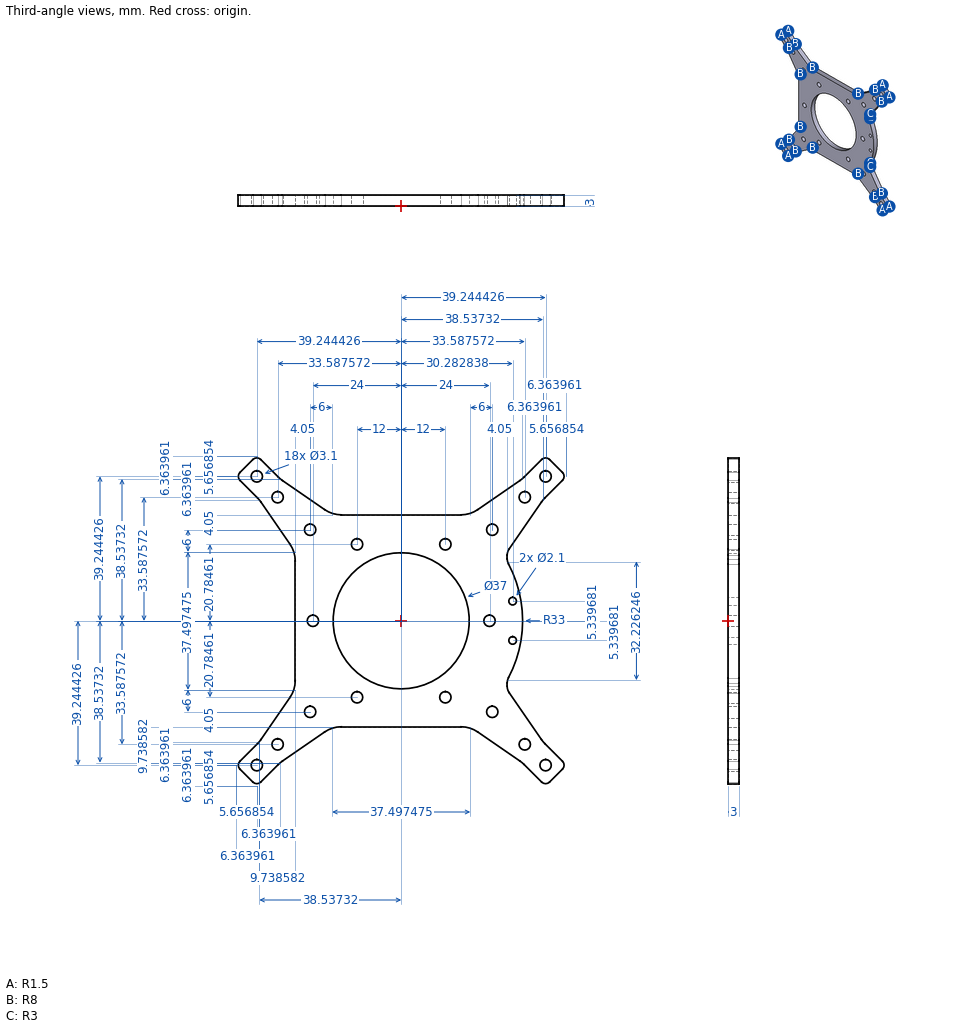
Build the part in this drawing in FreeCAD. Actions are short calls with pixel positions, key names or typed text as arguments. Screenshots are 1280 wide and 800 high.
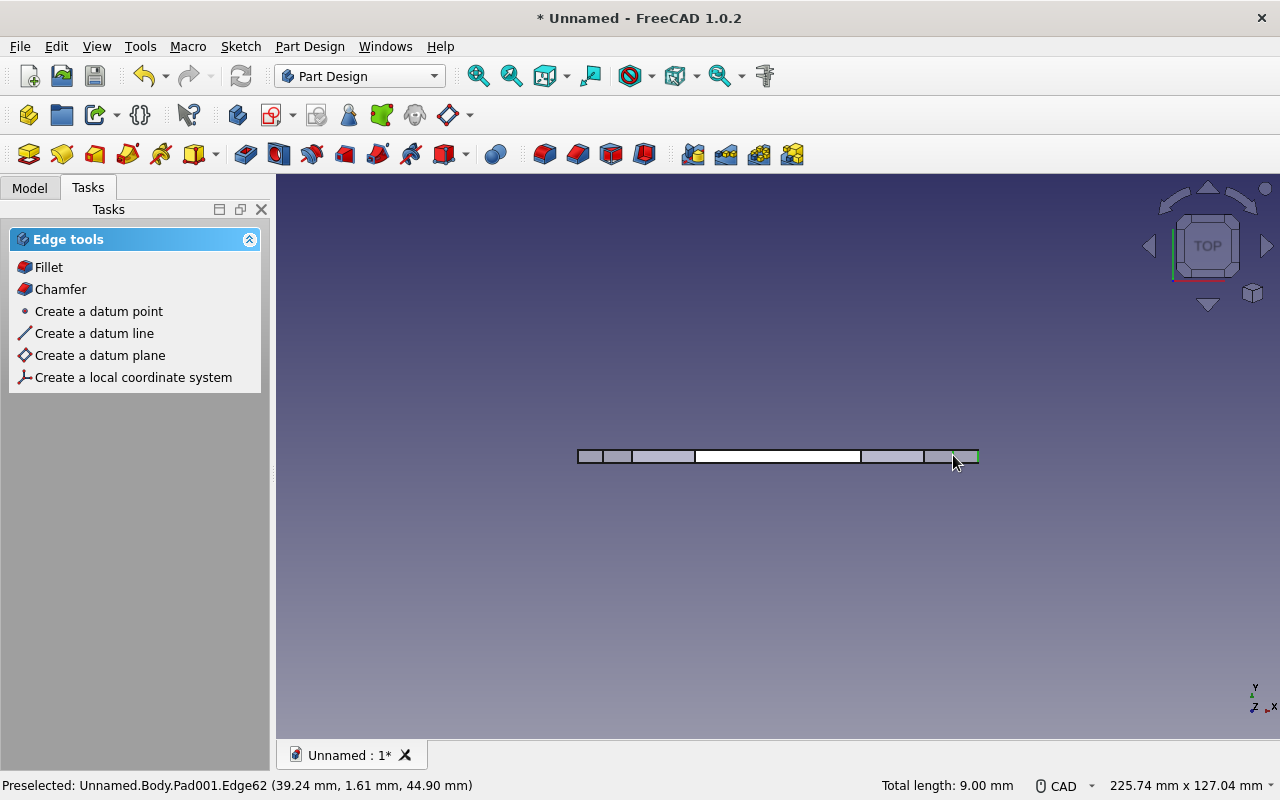
click(603, 455, ctrl)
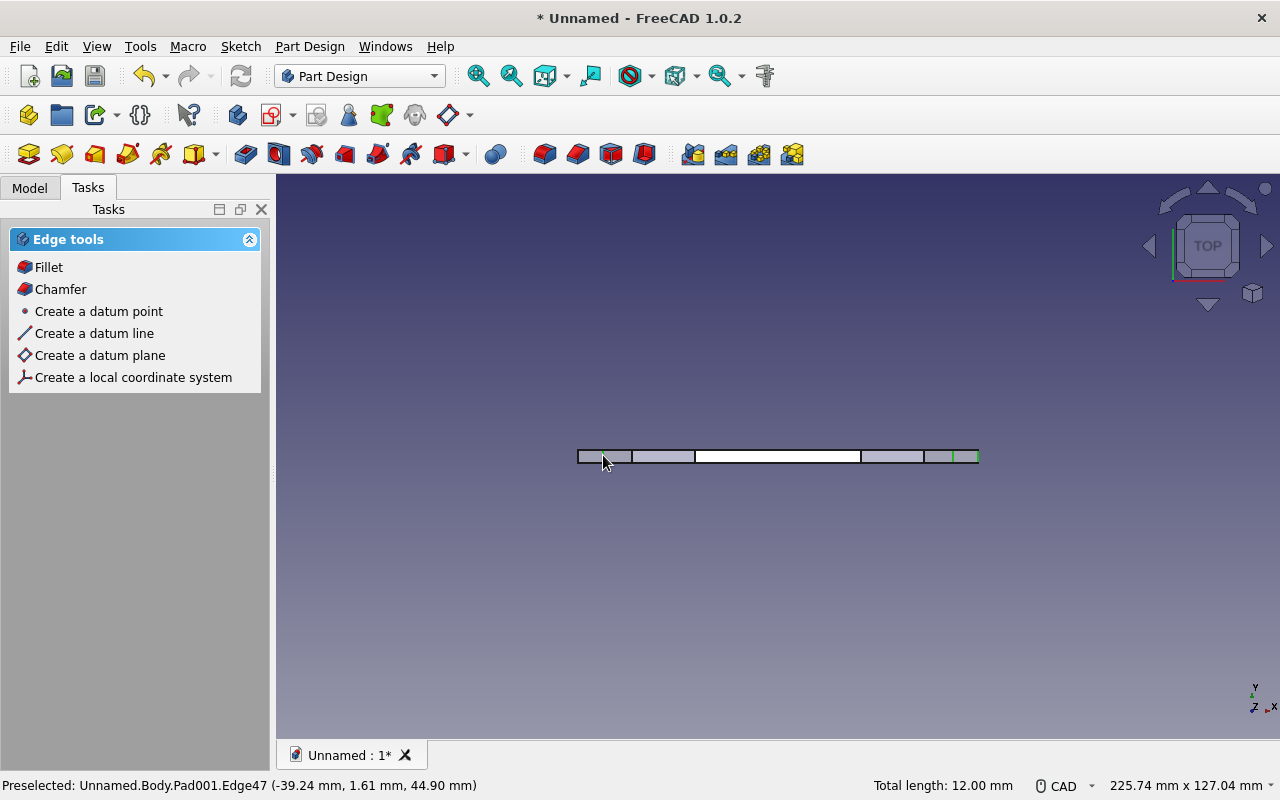
scroll(953, 455, up, 6)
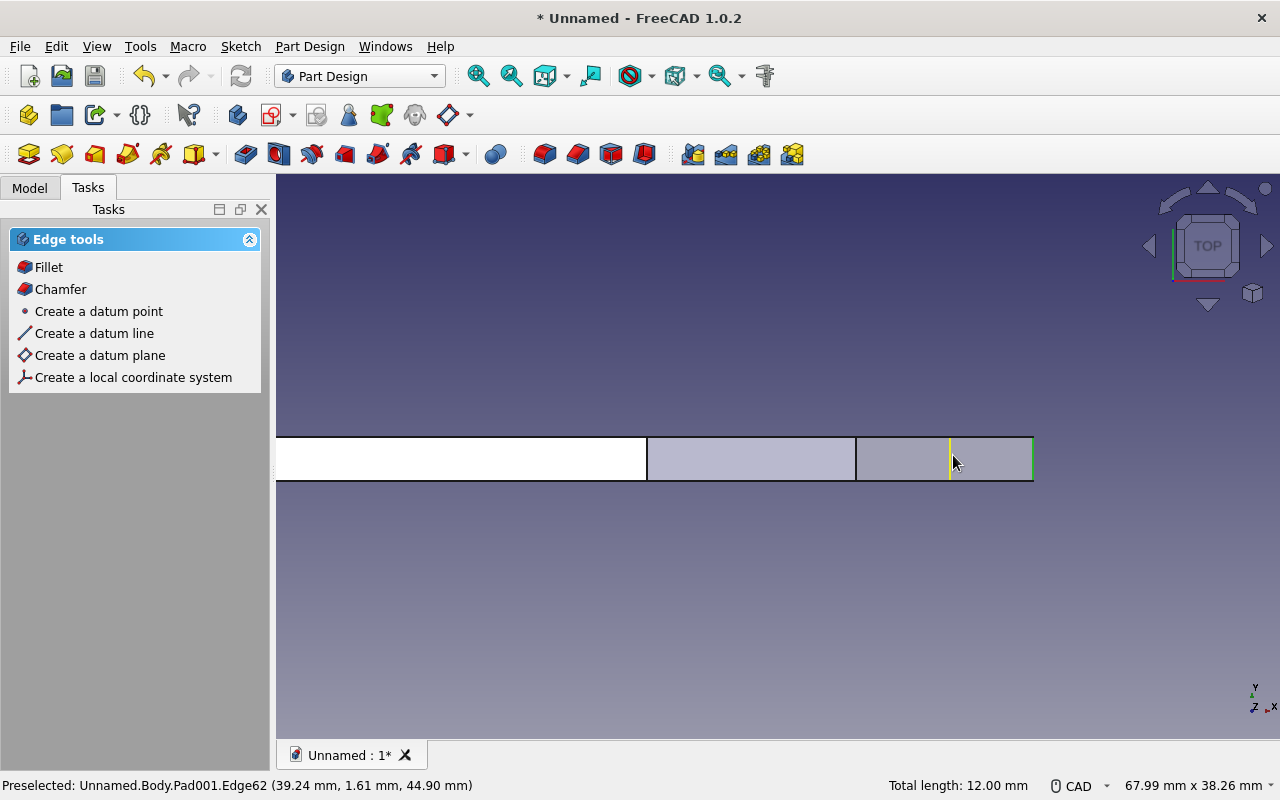
click(479, 76)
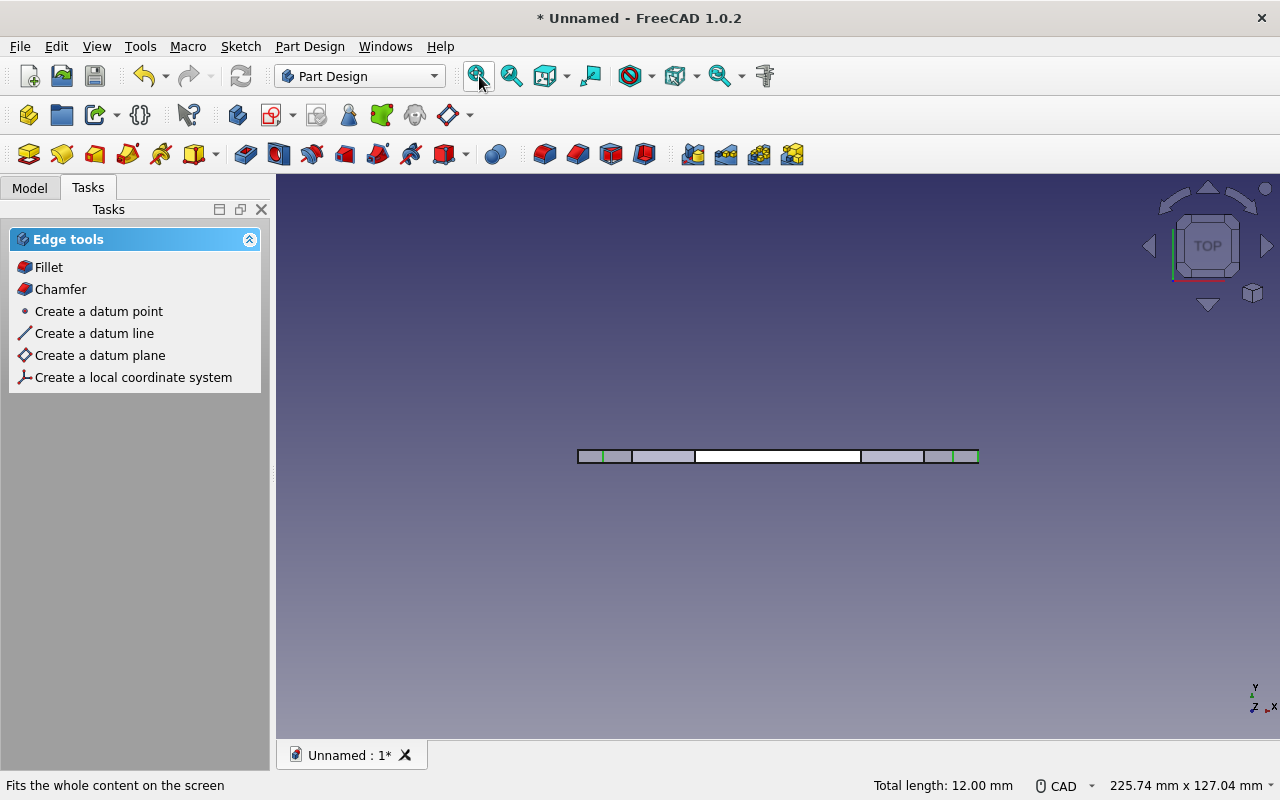
key(1)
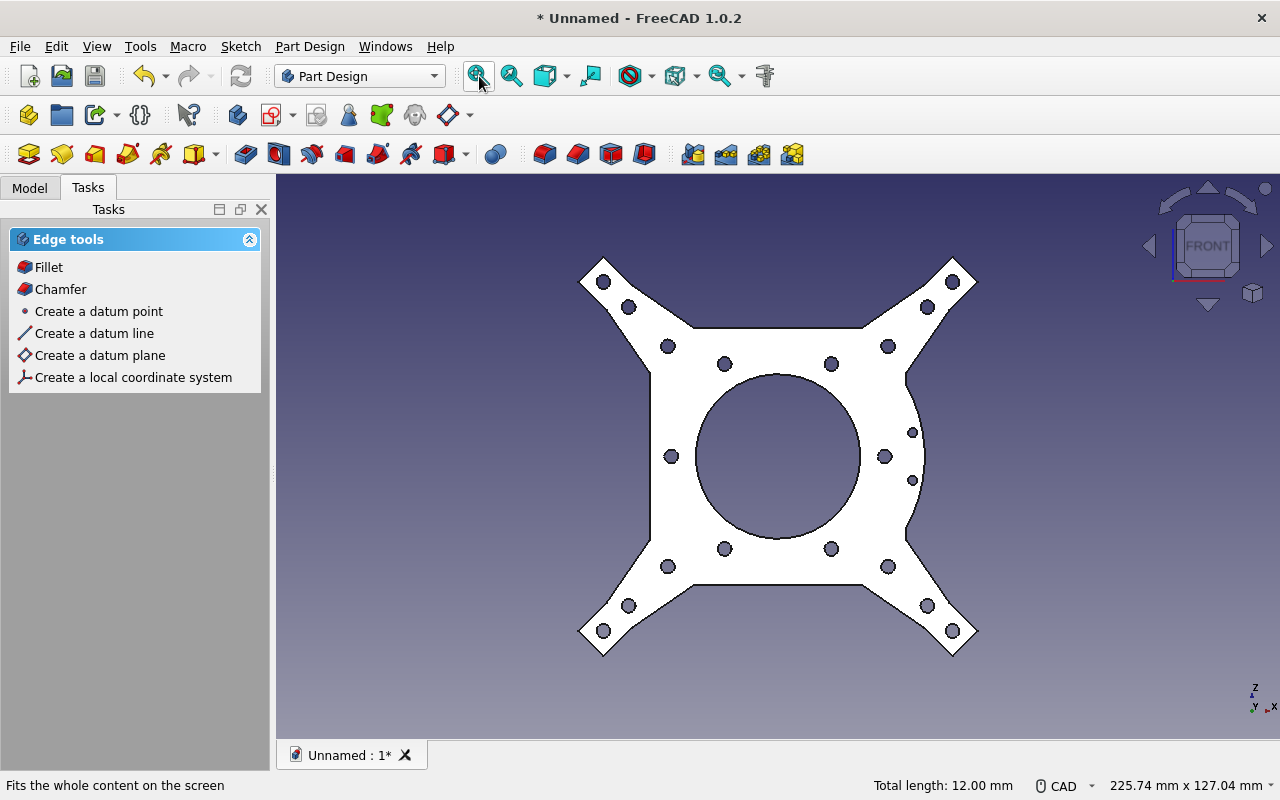
scroll(953, 655, up, 6)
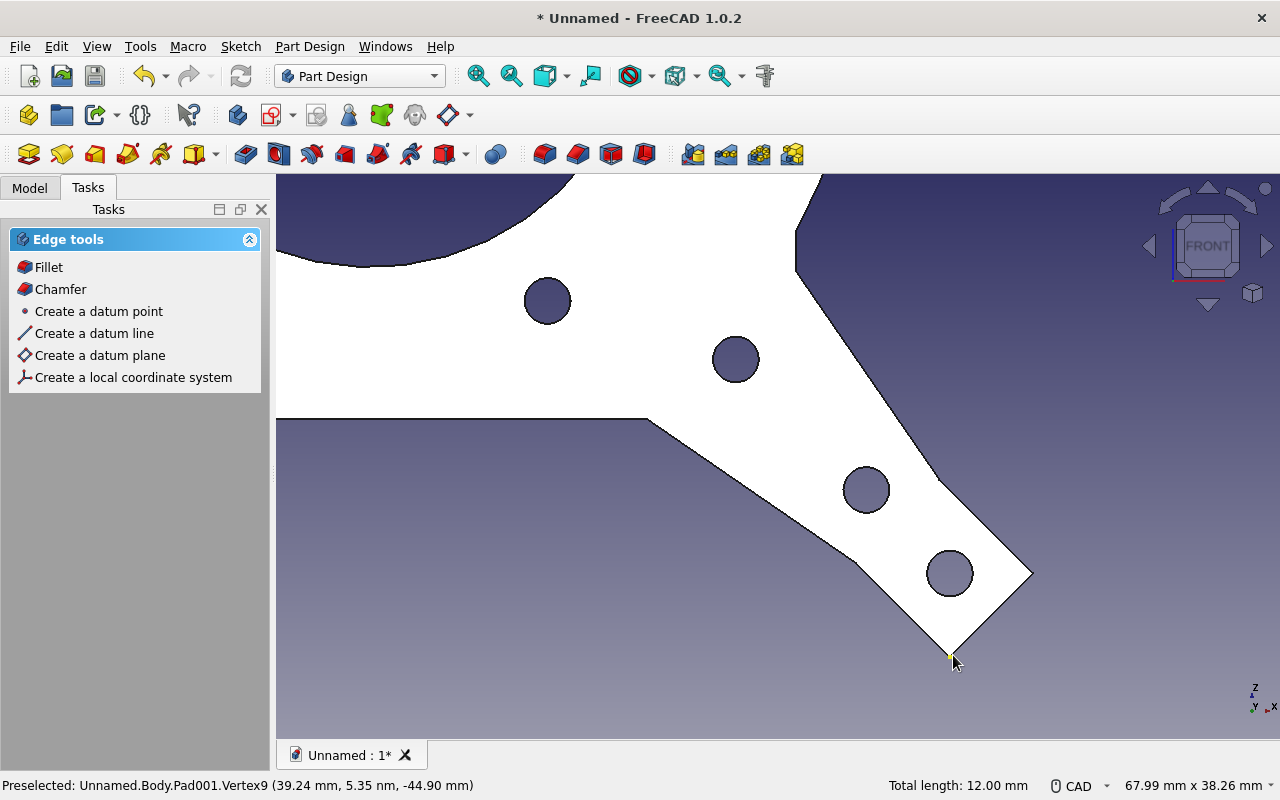
click(479, 76)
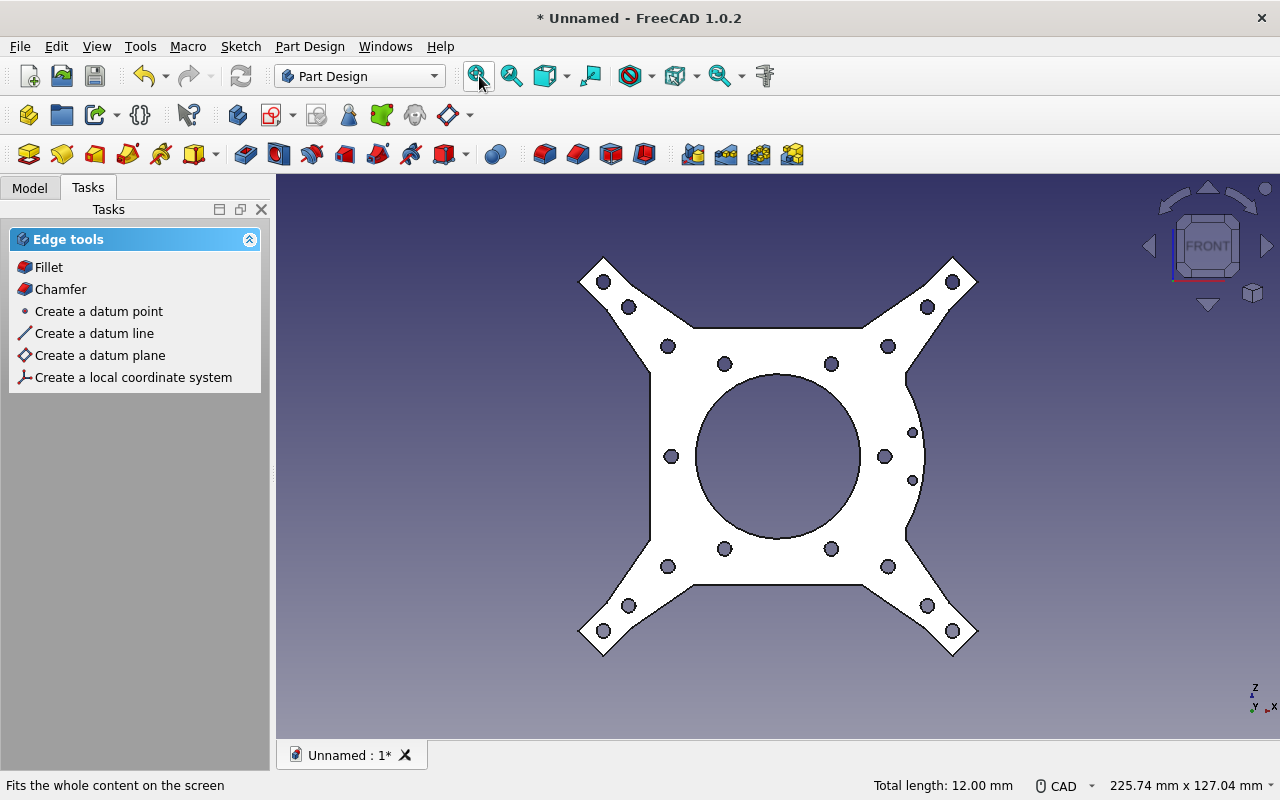
key(3)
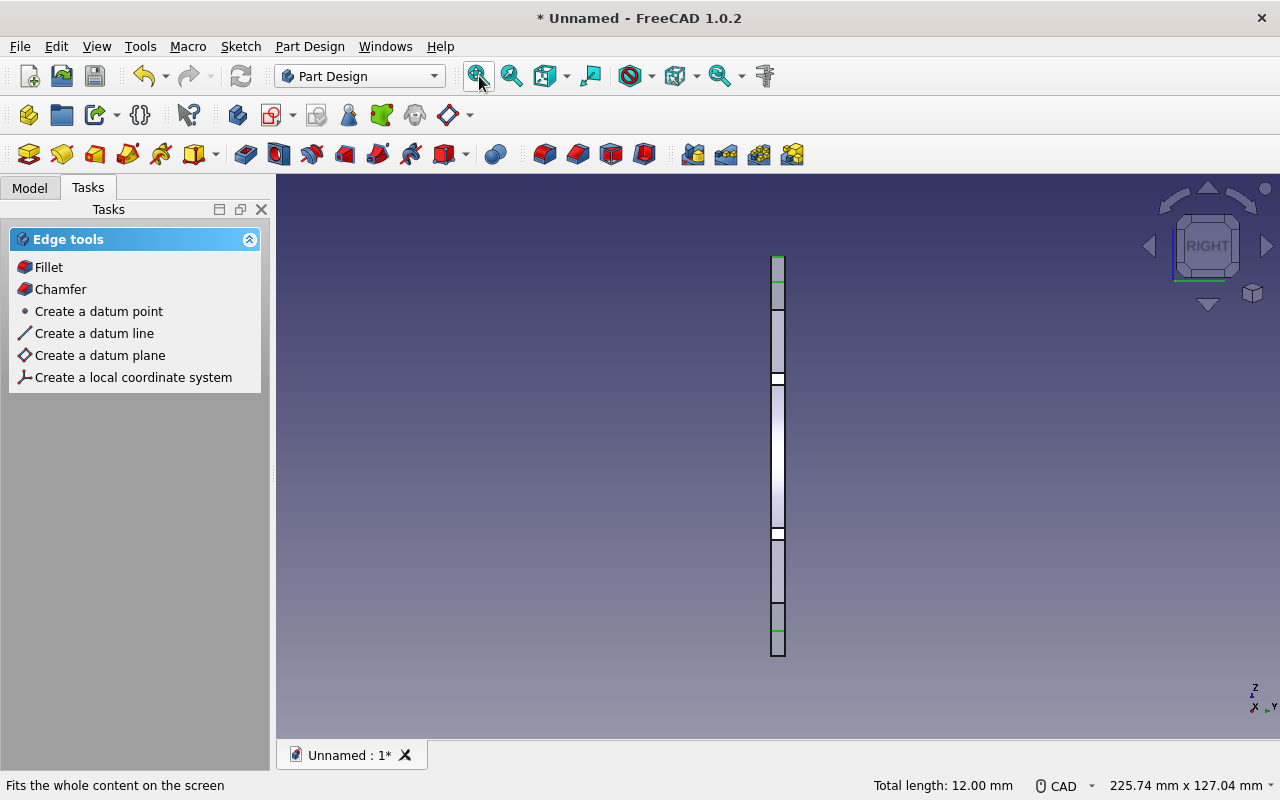
scroll(778, 655, up, 6)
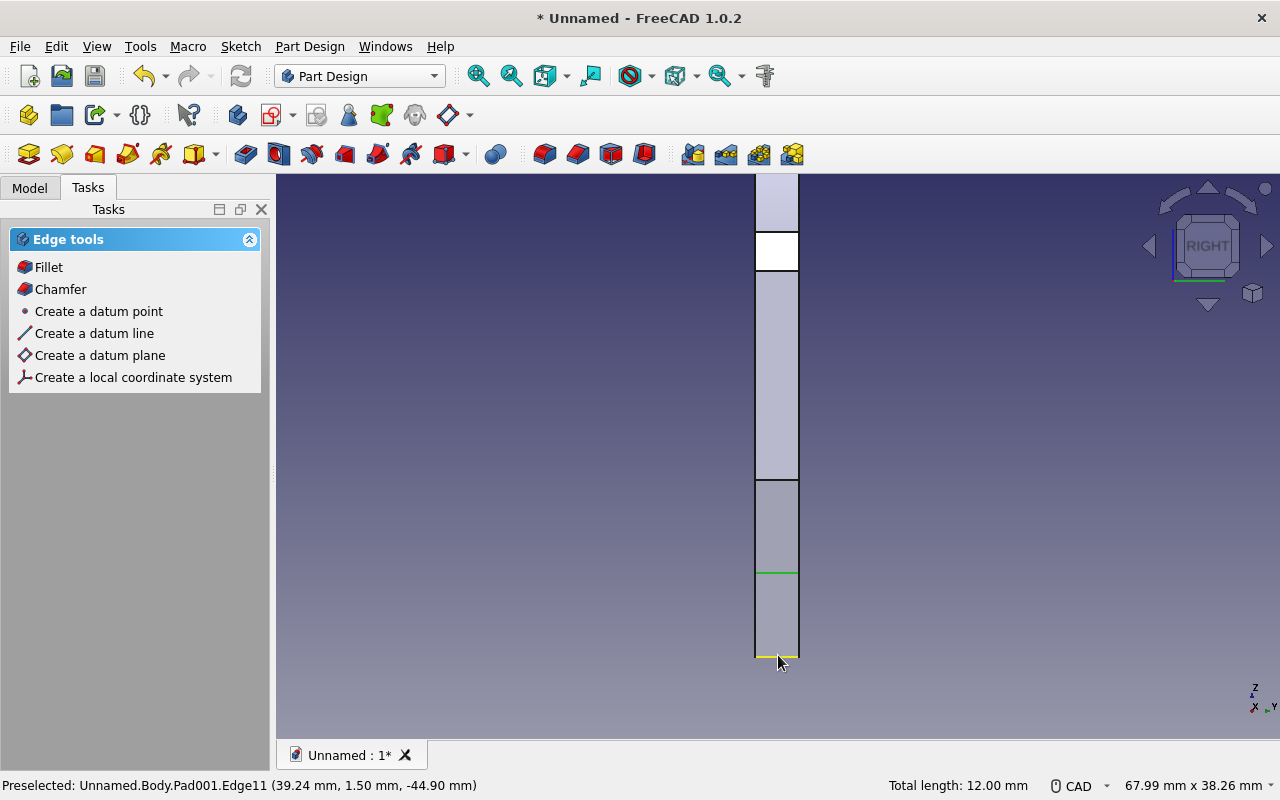
click(479, 76)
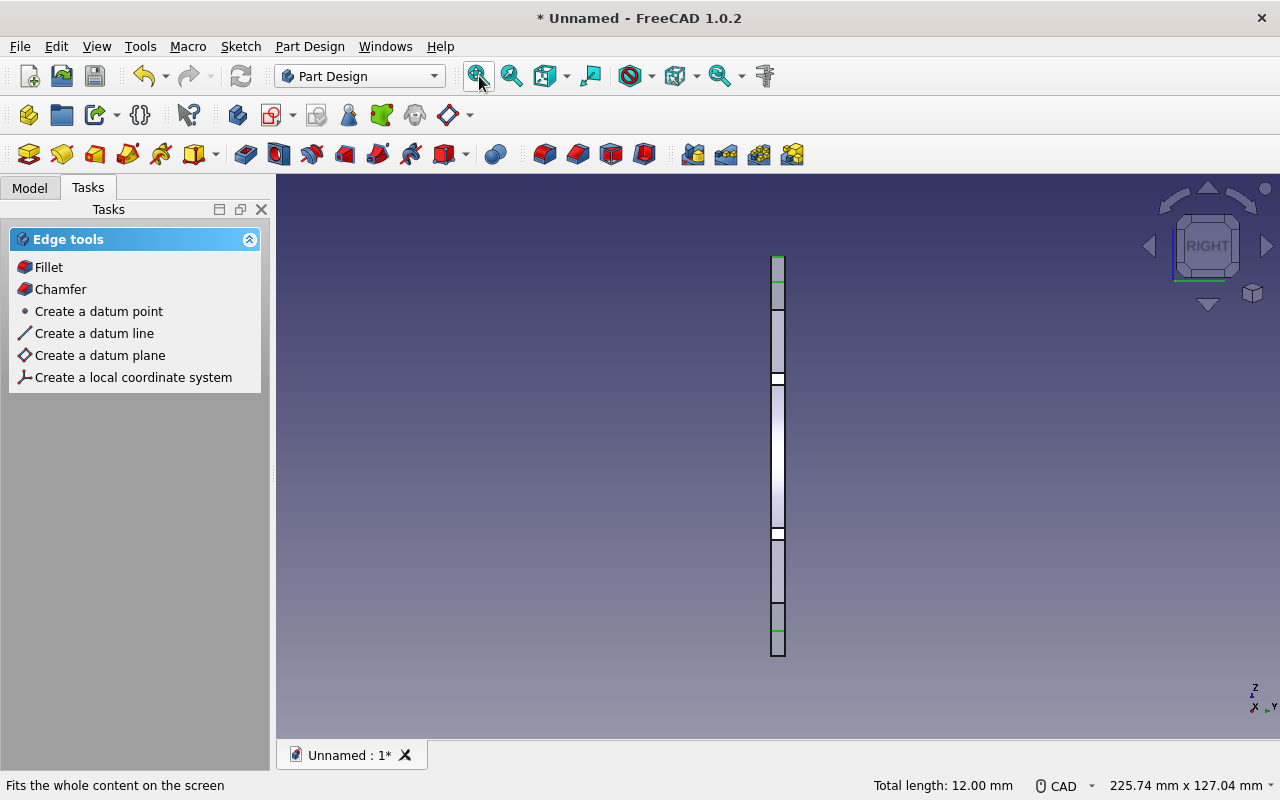
key(5)